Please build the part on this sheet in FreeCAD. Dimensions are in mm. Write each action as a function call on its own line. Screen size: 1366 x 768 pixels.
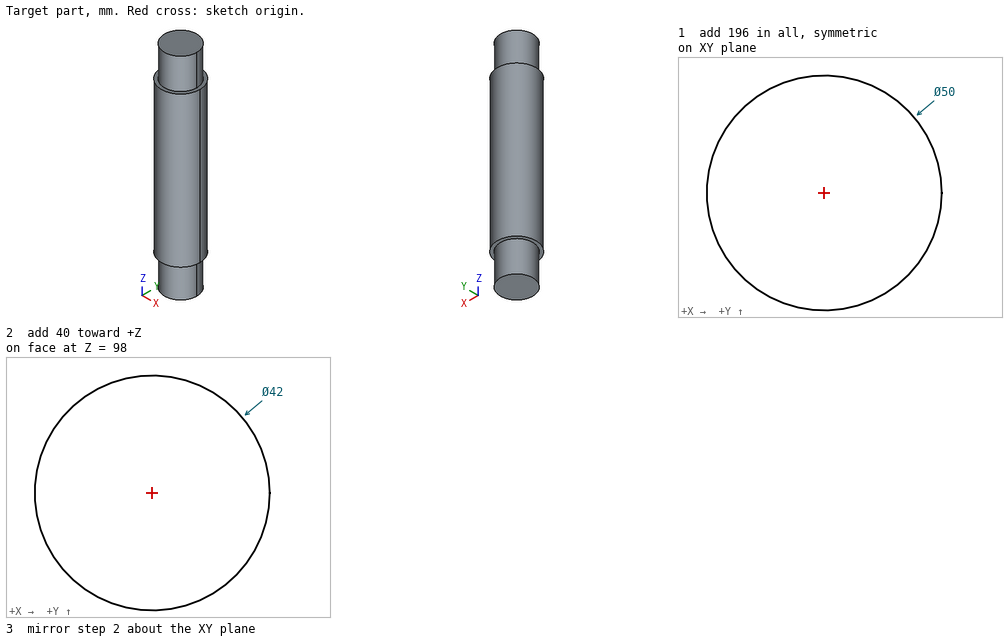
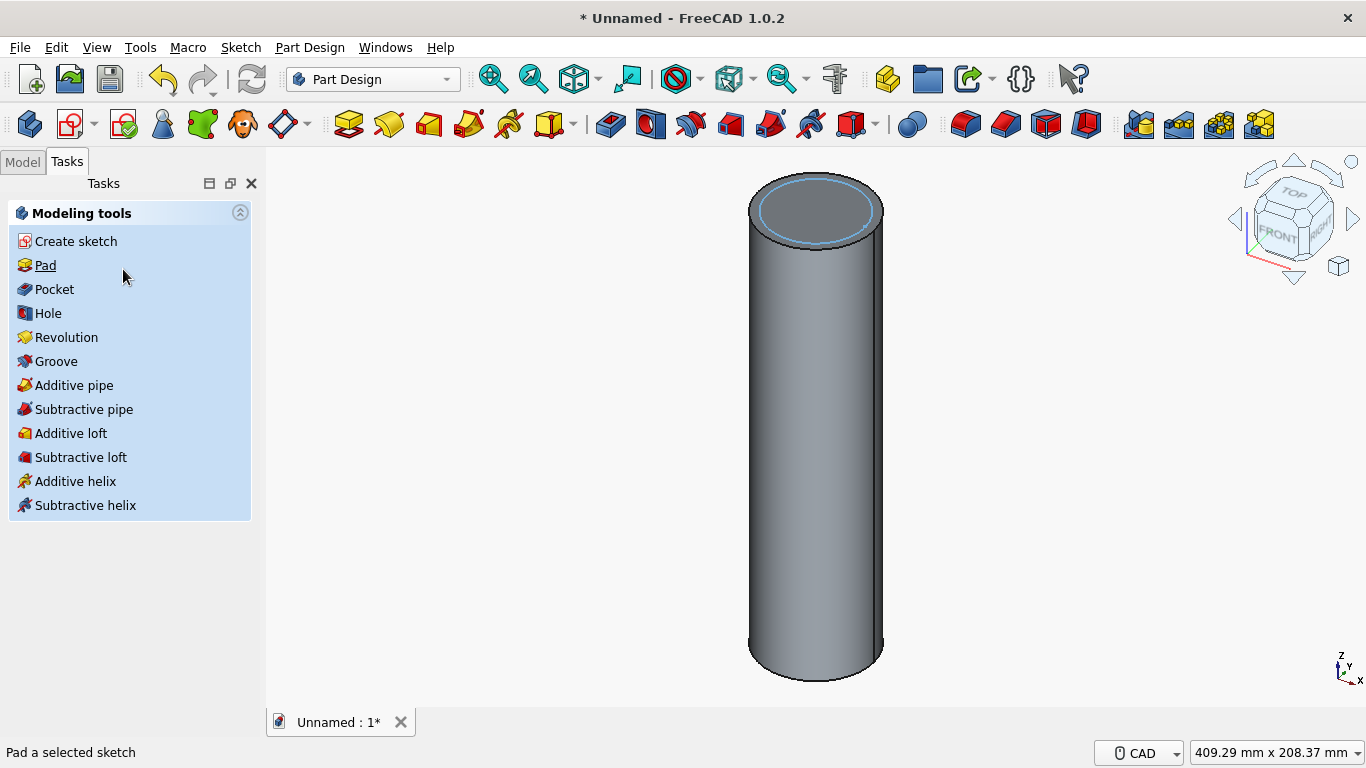
click(350, 124)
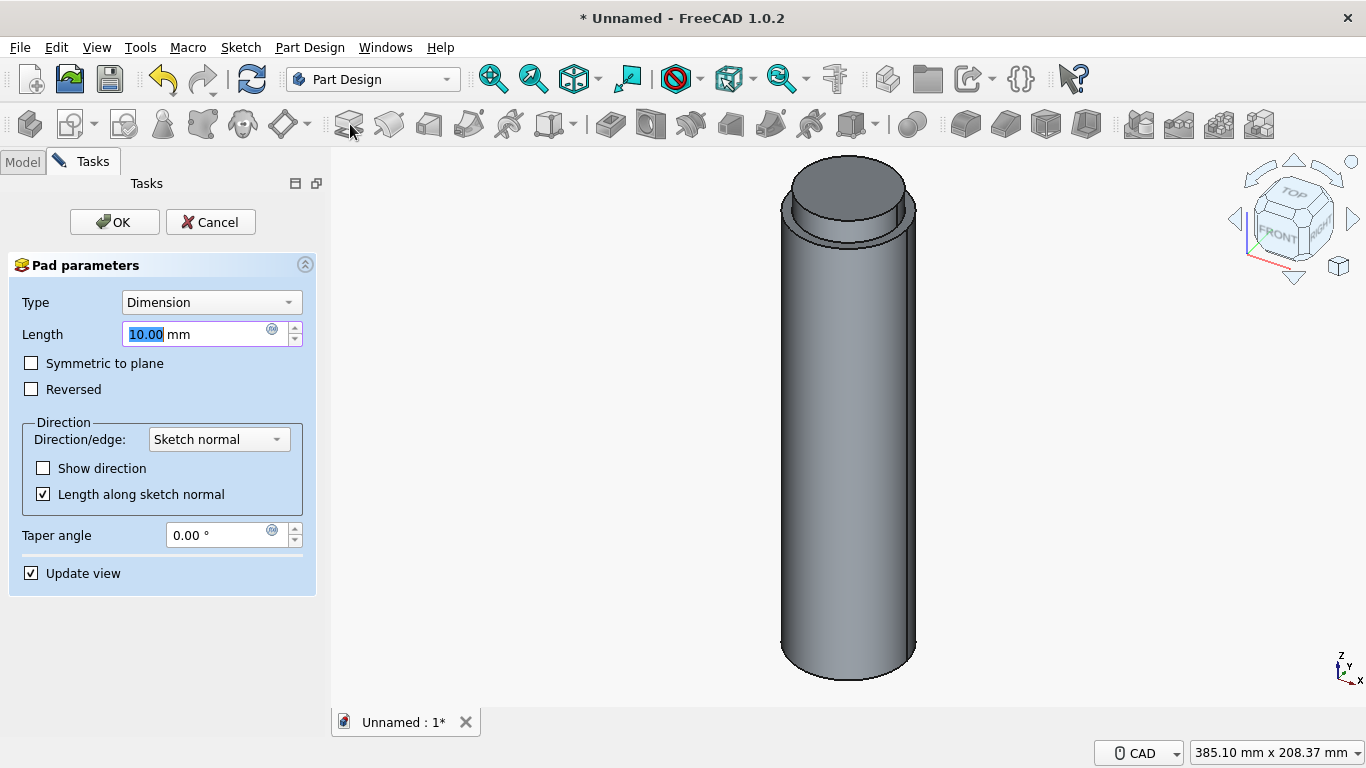
text(40)
key(Tab)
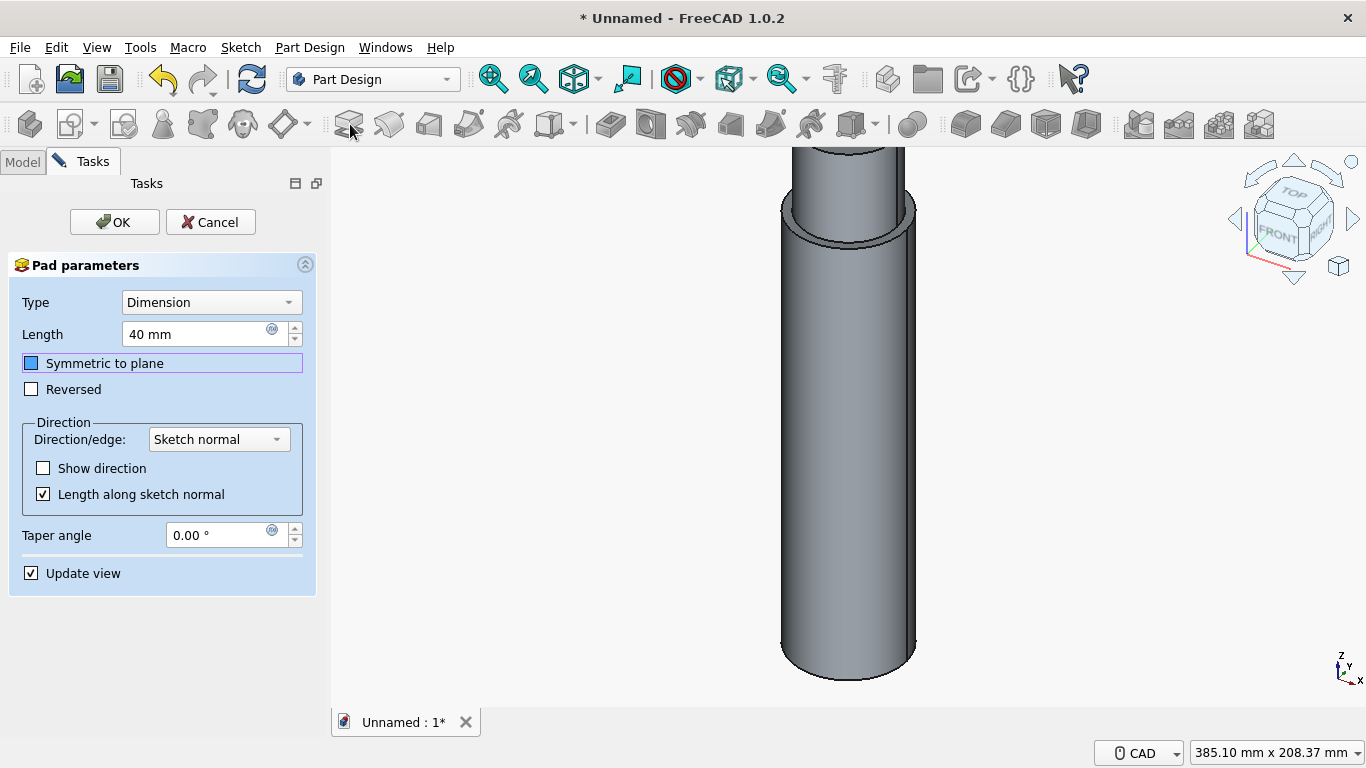
click(115, 222)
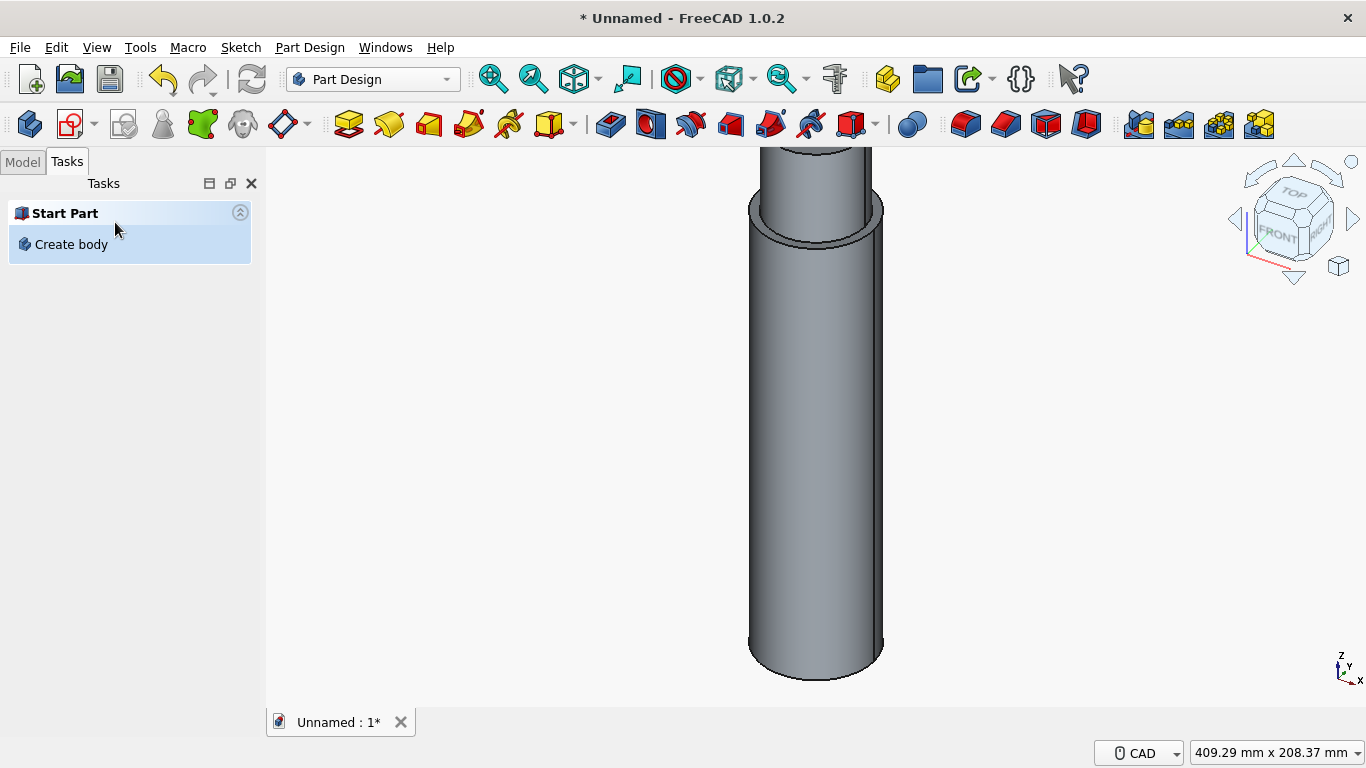
click(494, 80)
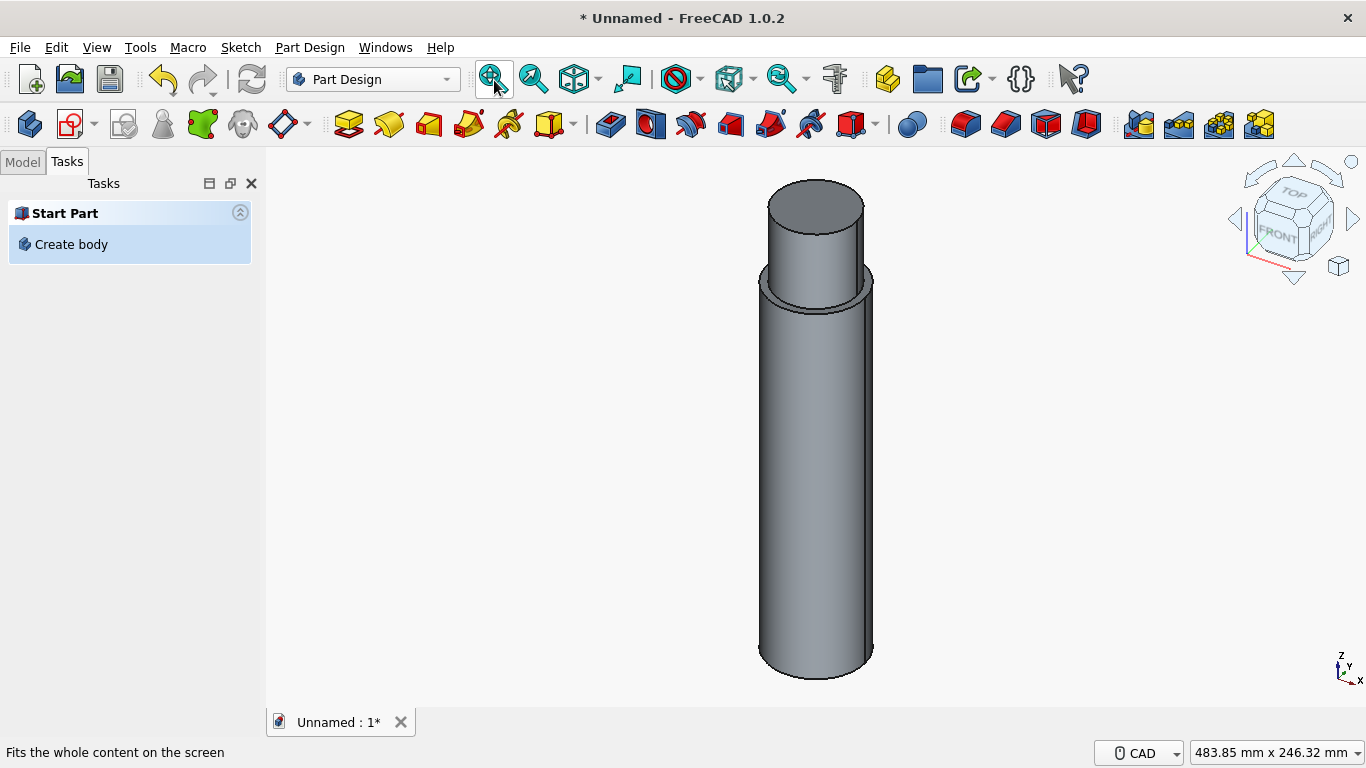
click(23, 161)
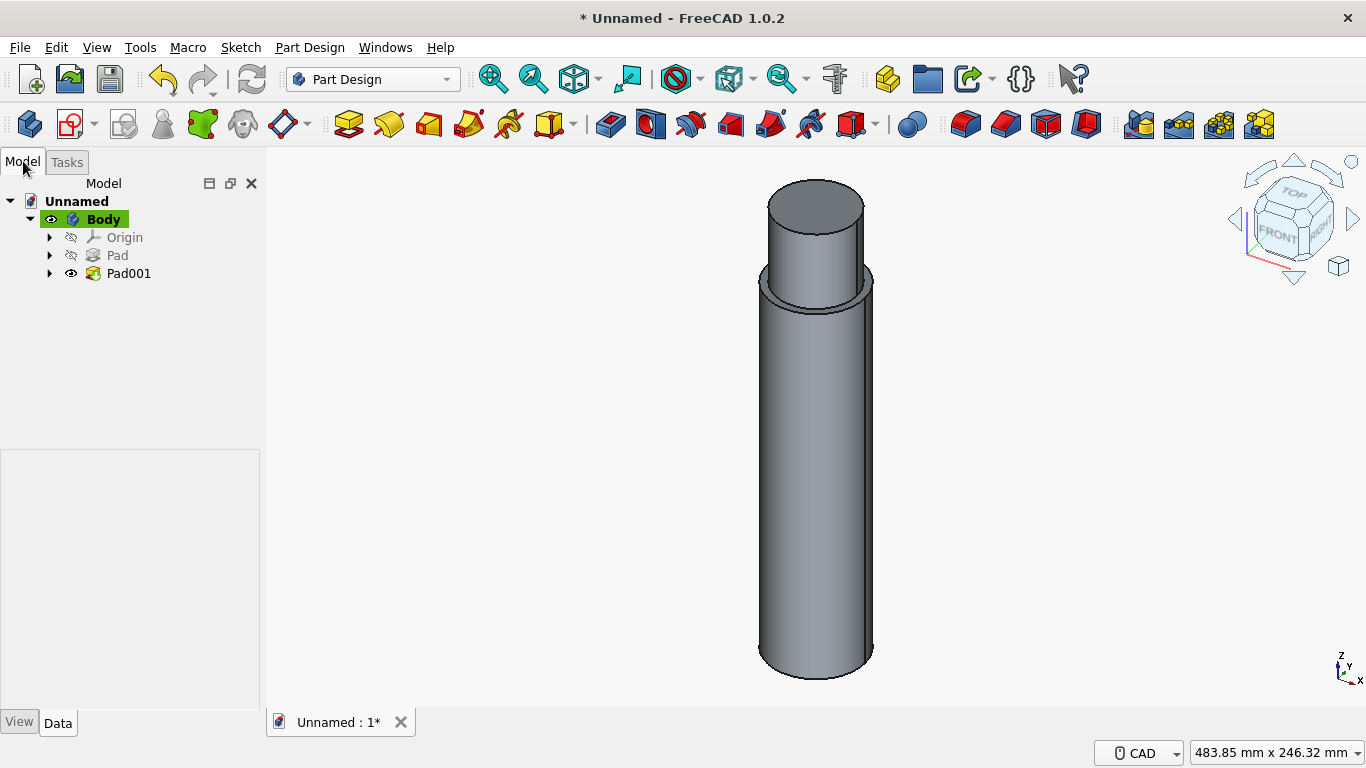
click(116, 273)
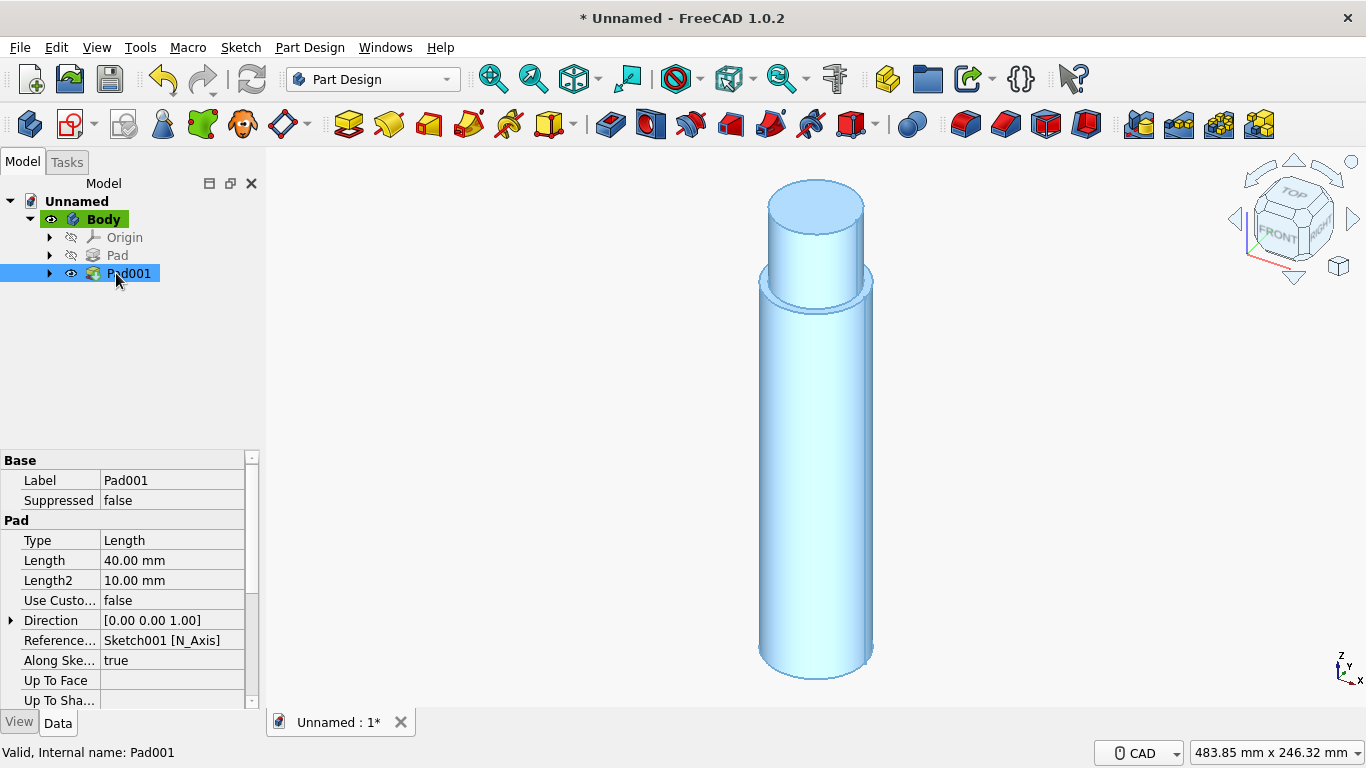
click(1140, 124)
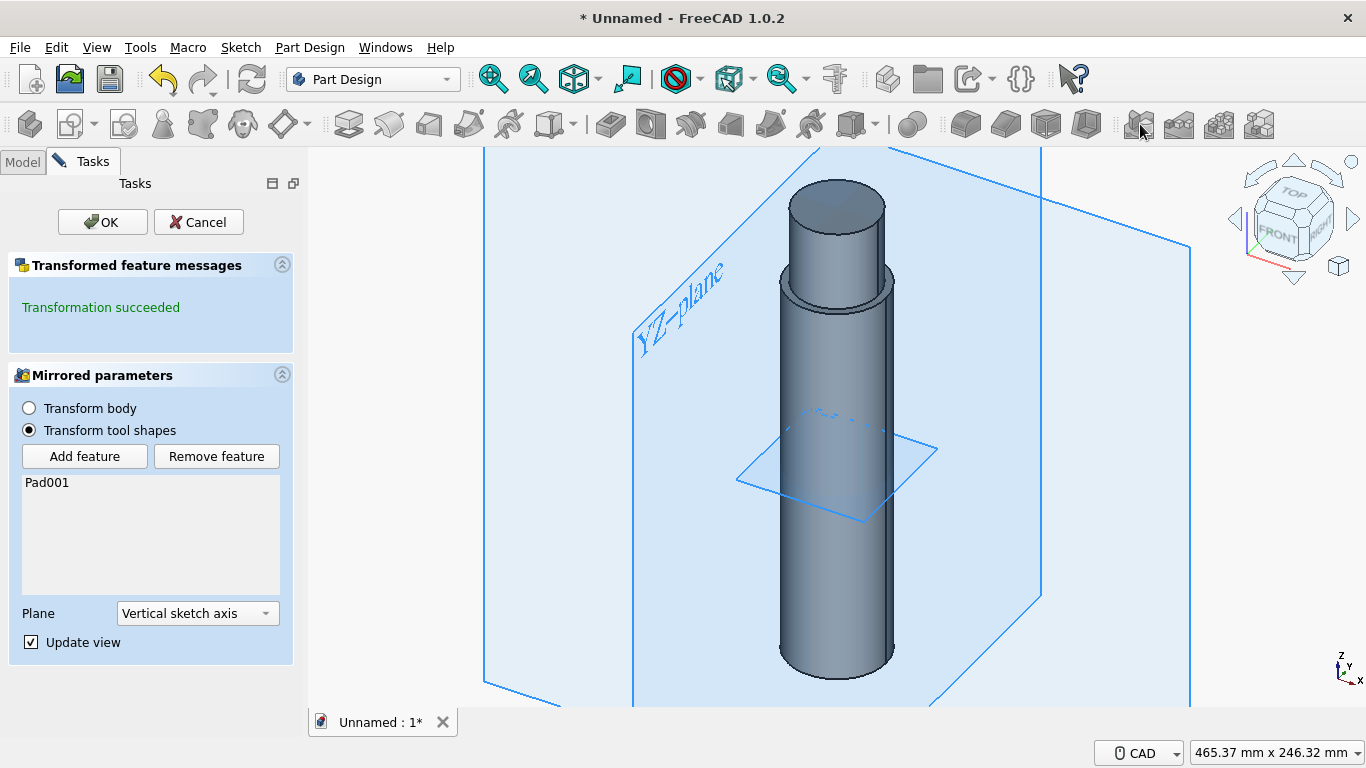
click(198, 614)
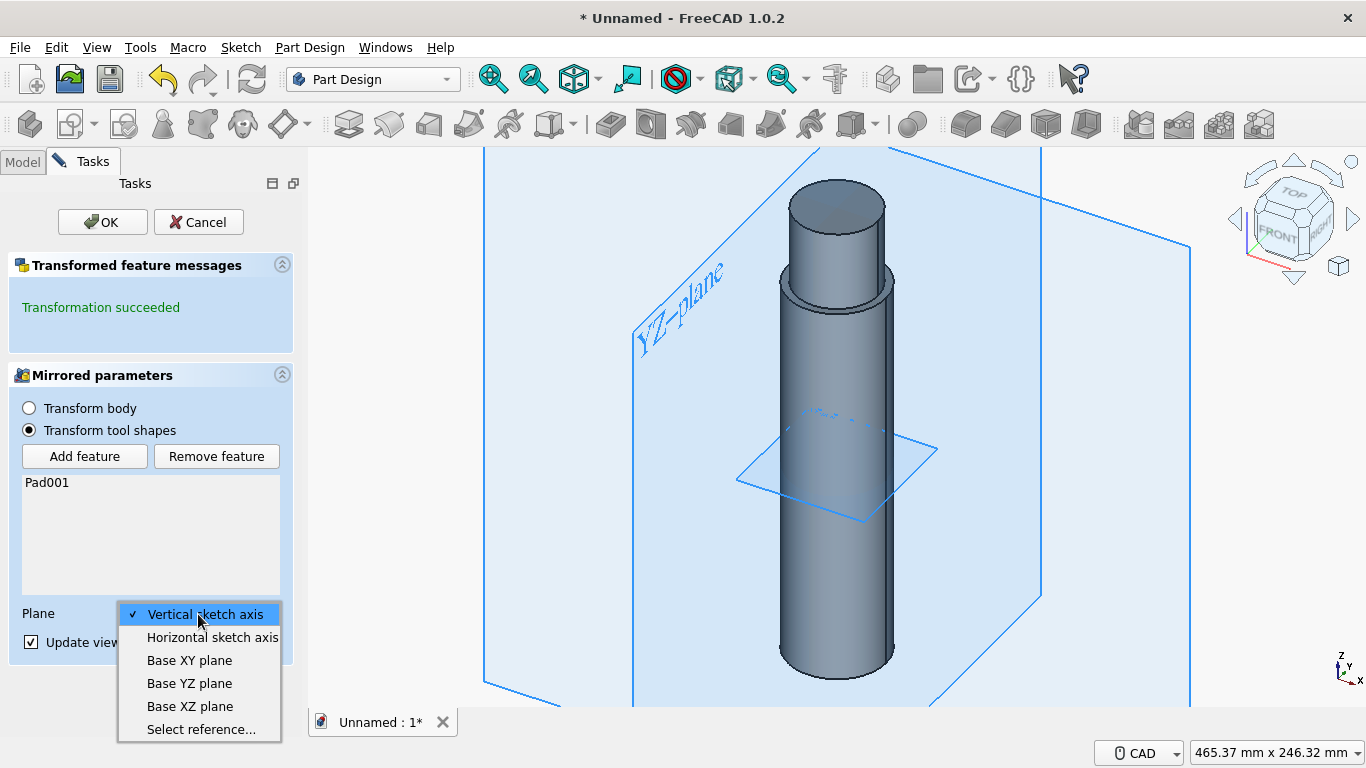
click(198, 660)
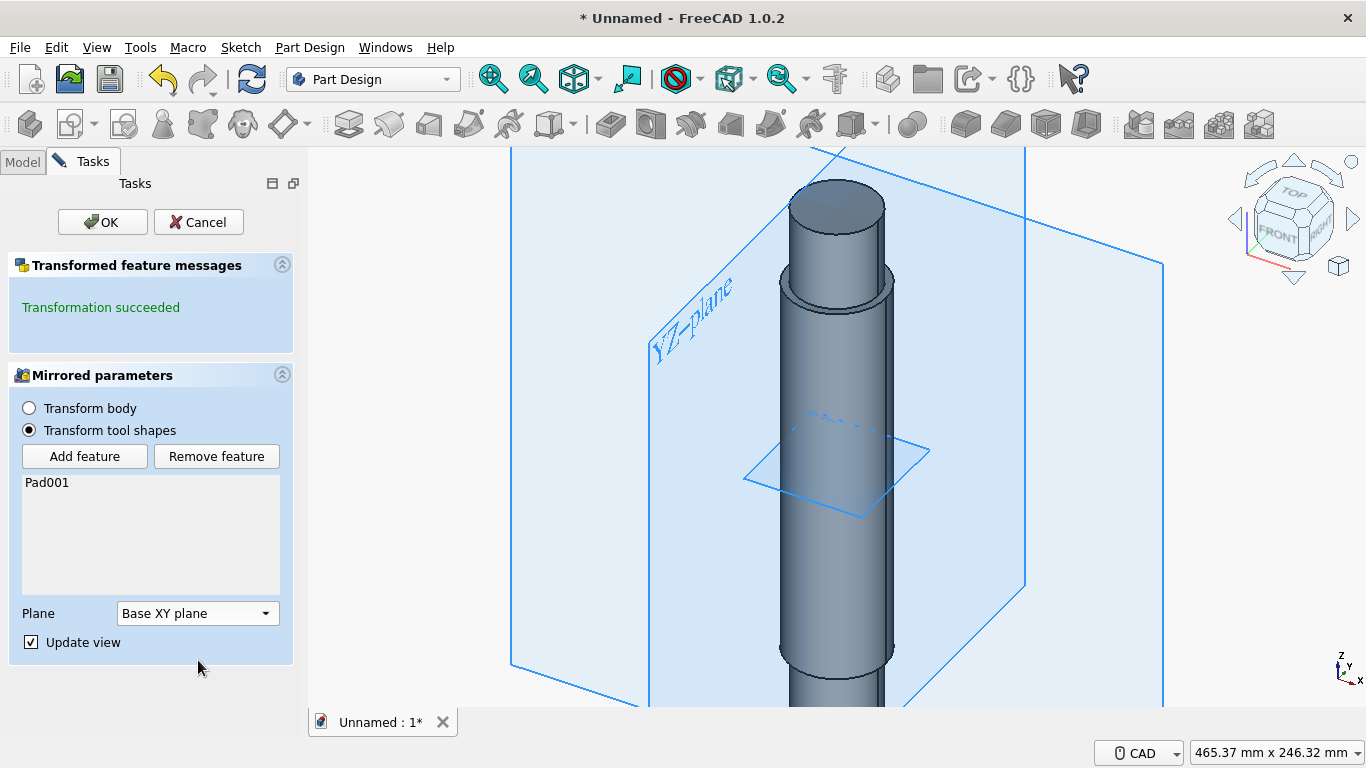
click(103, 222)